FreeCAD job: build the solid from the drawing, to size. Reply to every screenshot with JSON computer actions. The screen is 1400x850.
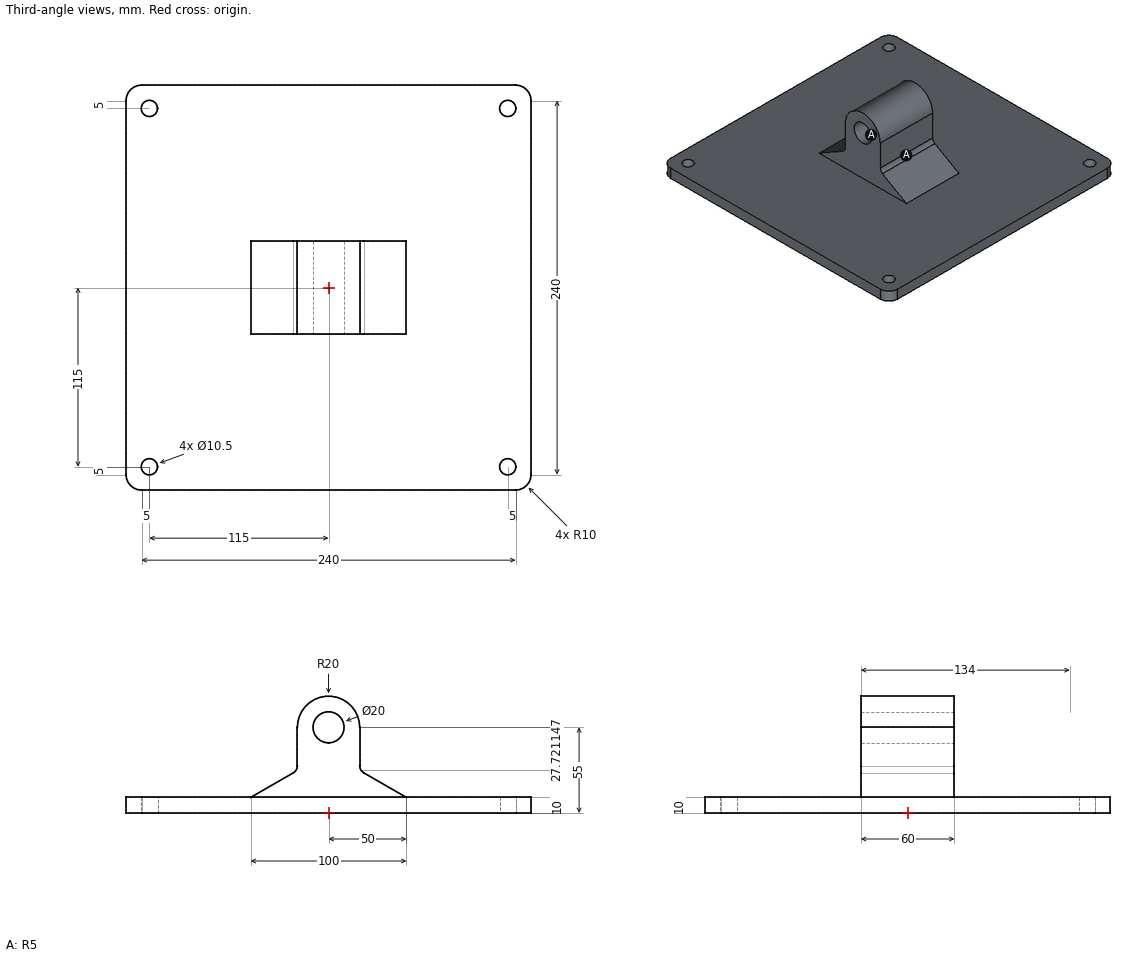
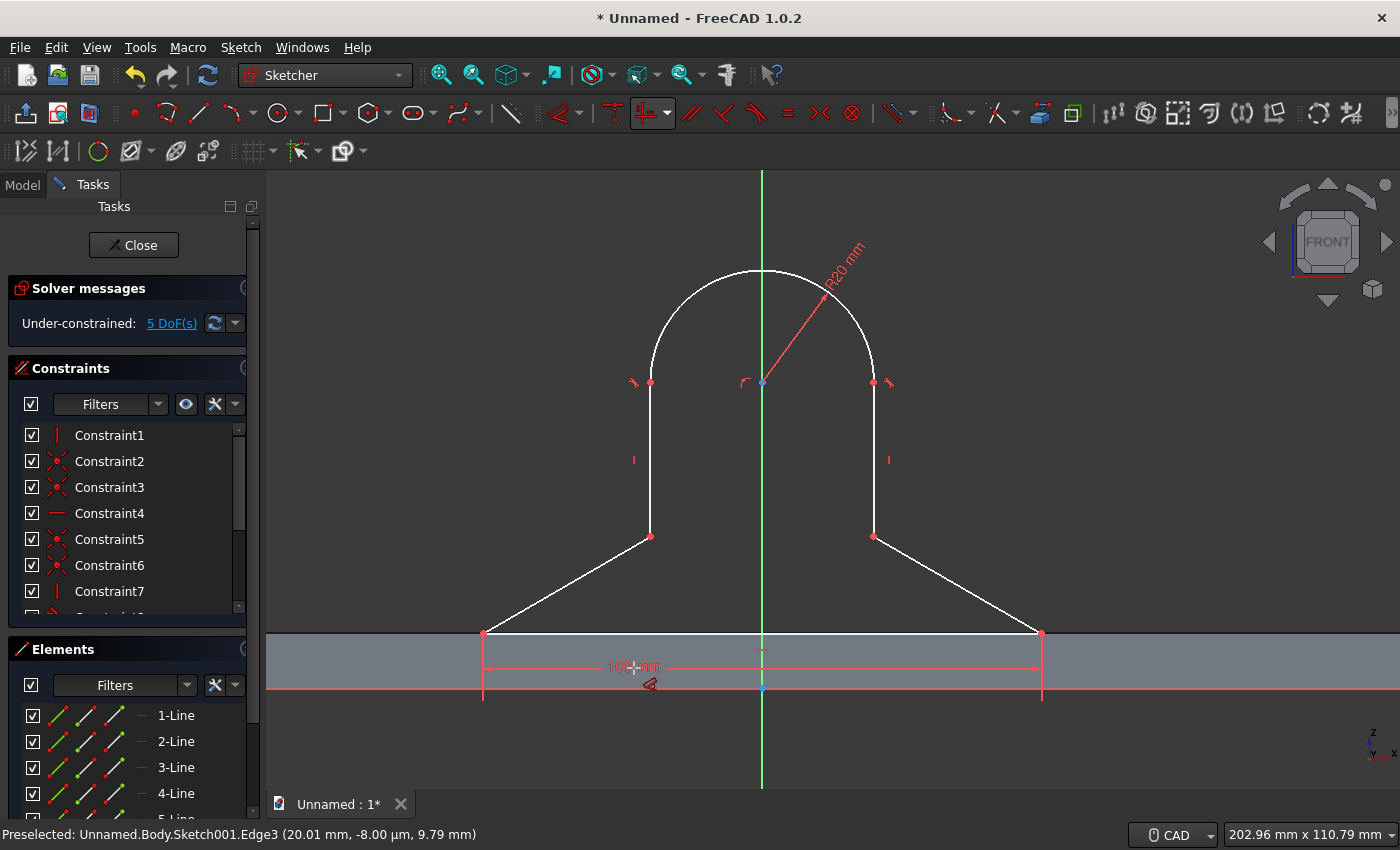
{"action": "left_click", "coordinate": [874, 382]}
{"action": "left_click", "coordinate": [908, 536]}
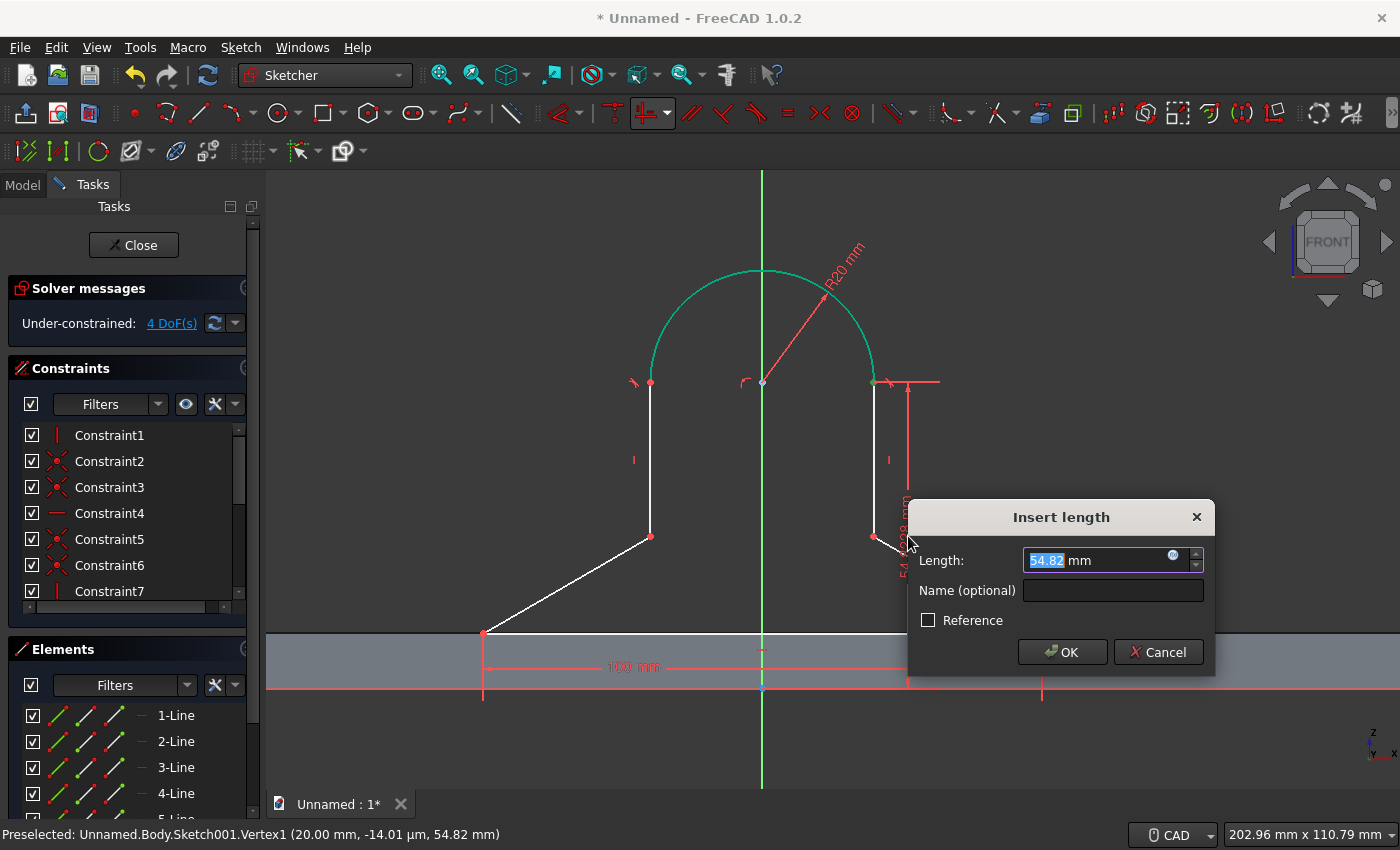
{"action": "type", "text": "55"}
{"action": "key", "text": "Return"}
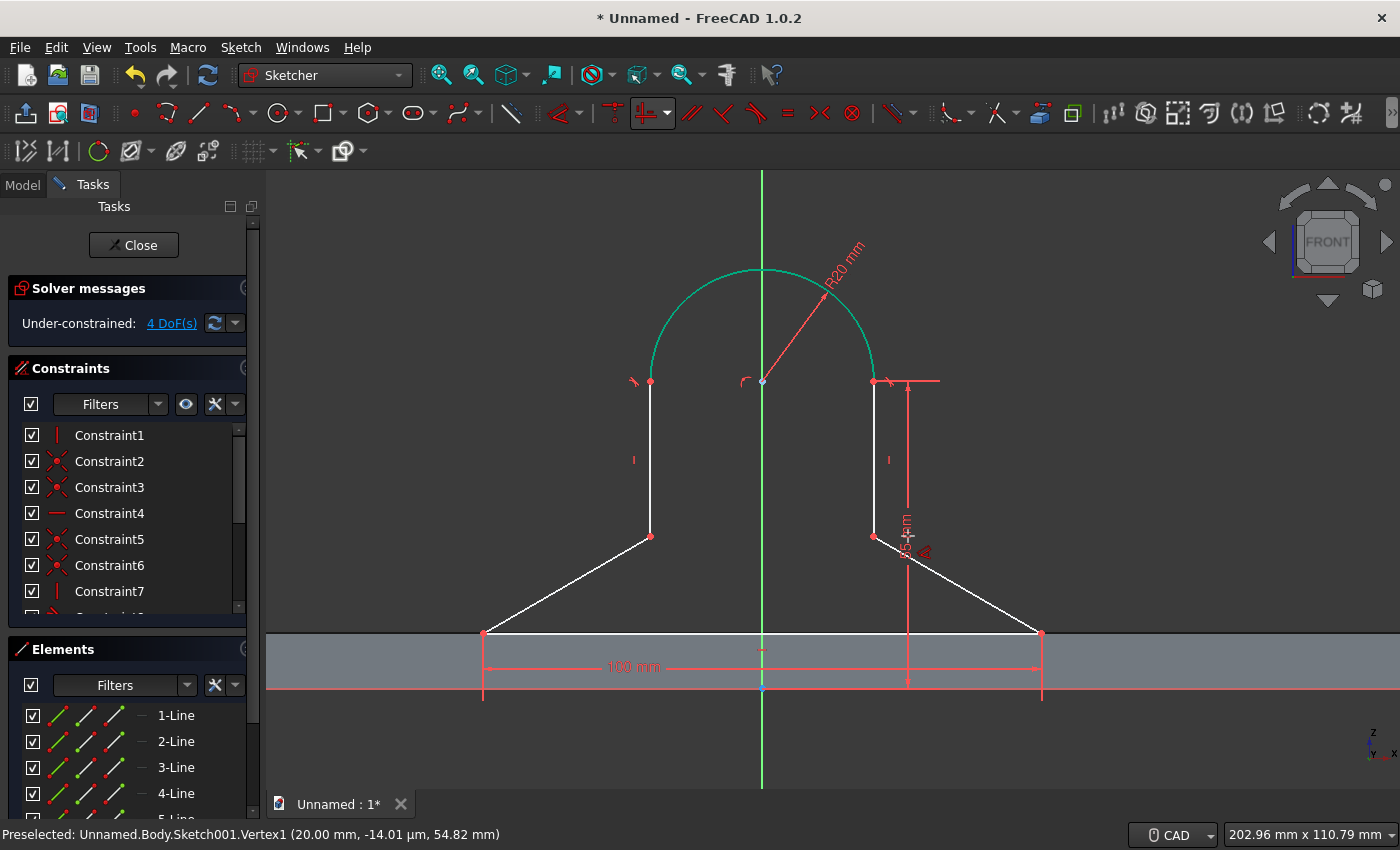
{"action": "left_click", "coordinate": [1042, 634]}
{"action": "left_click", "coordinate": [902, 723]}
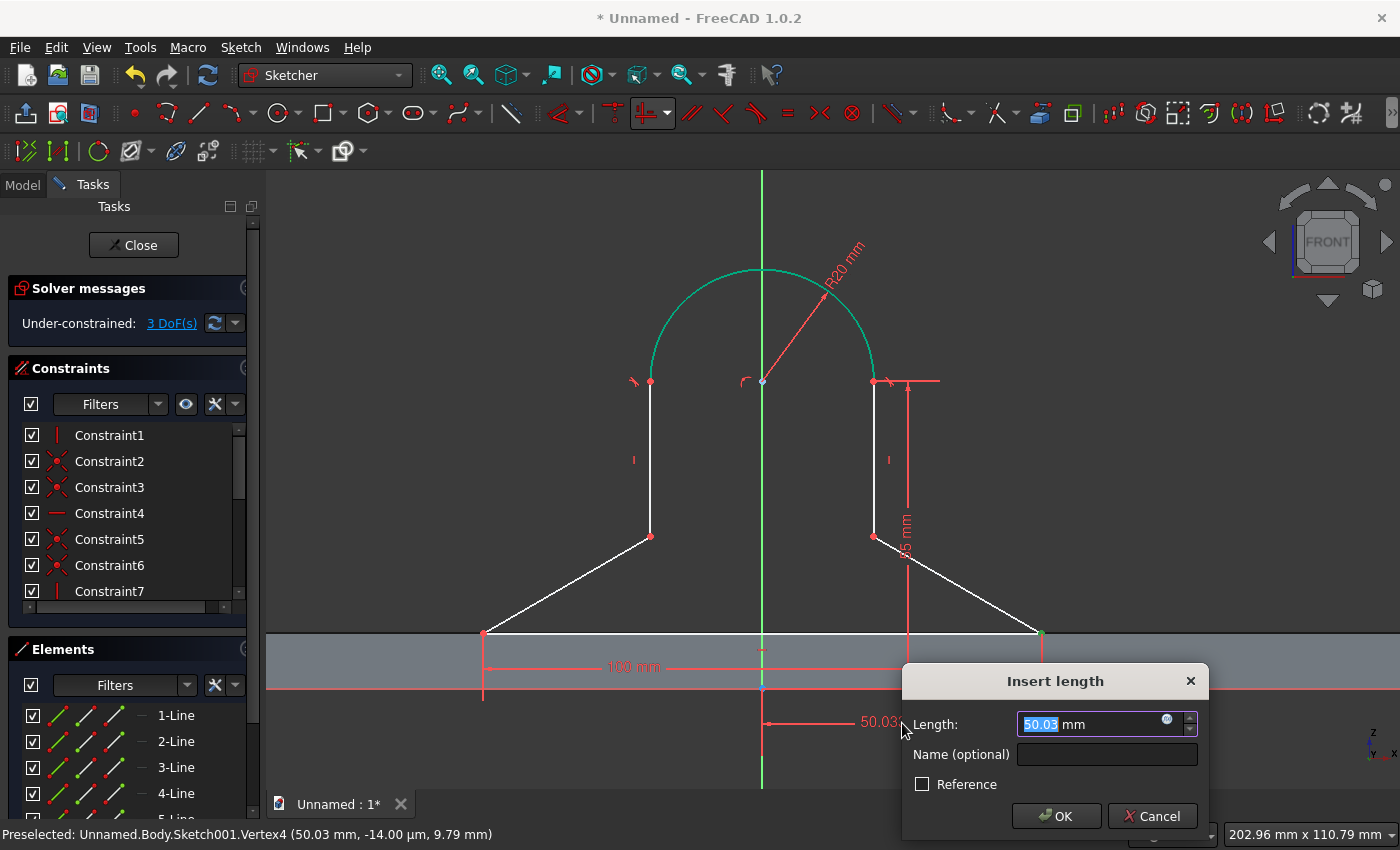
{"action": "type", "text": "50"}
{"action": "key", "text": "Return"}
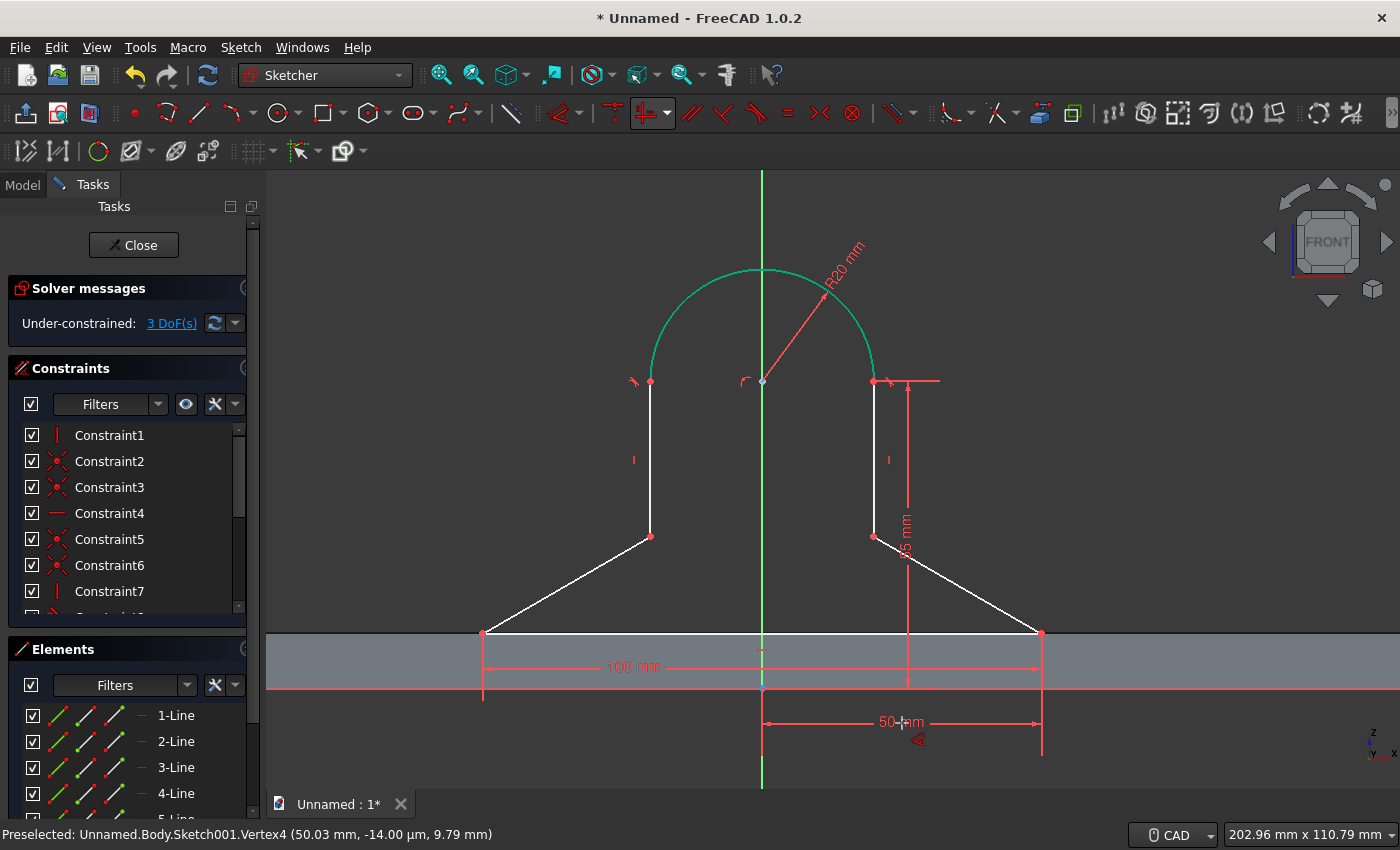
{"action": "left_click", "coordinate": [1042, 634]}
{"action": "left_click", "coordinate": [1076, 661]}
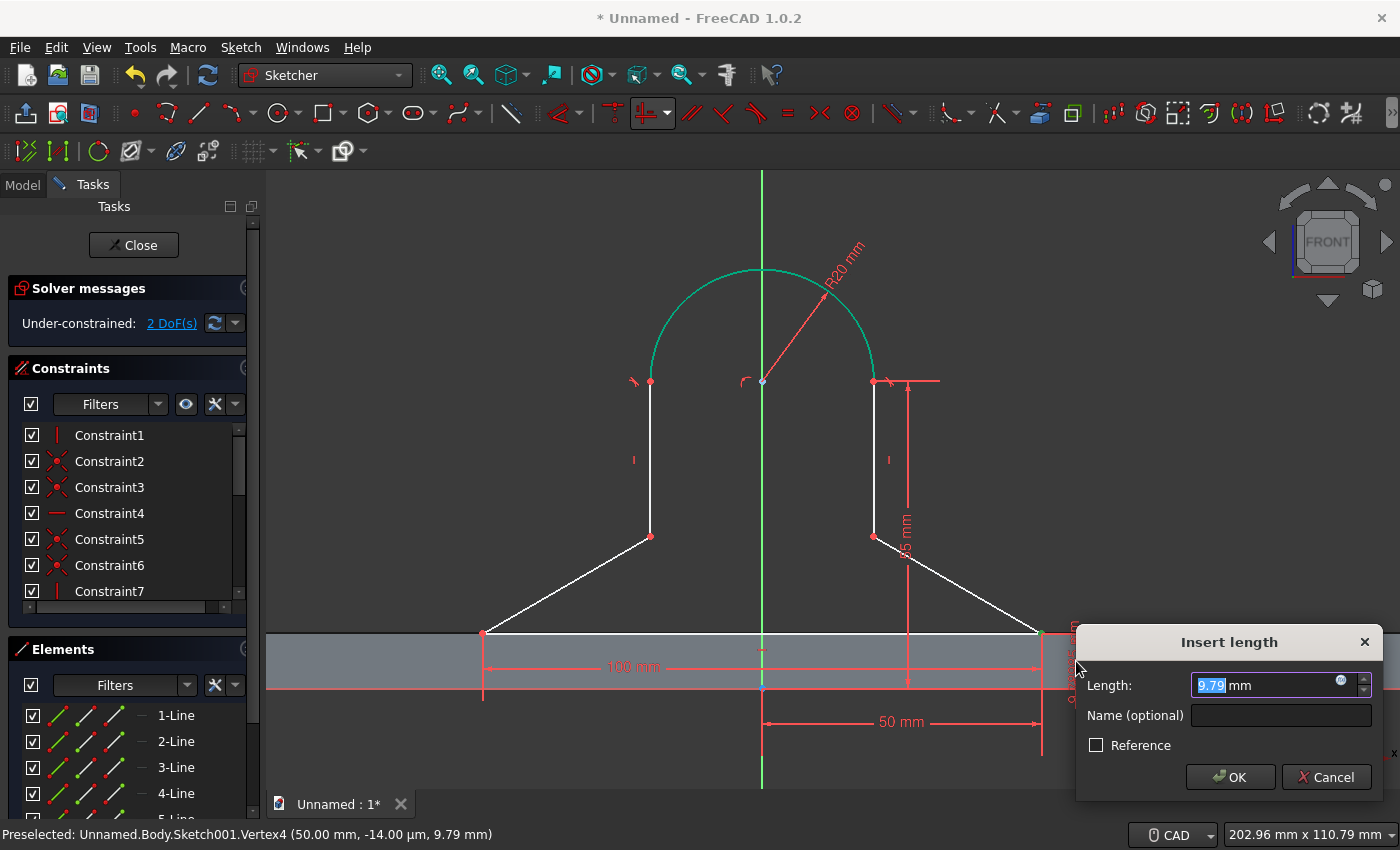
{"action": "type", "text": "10"}
{"action": "key", "text": "Return"}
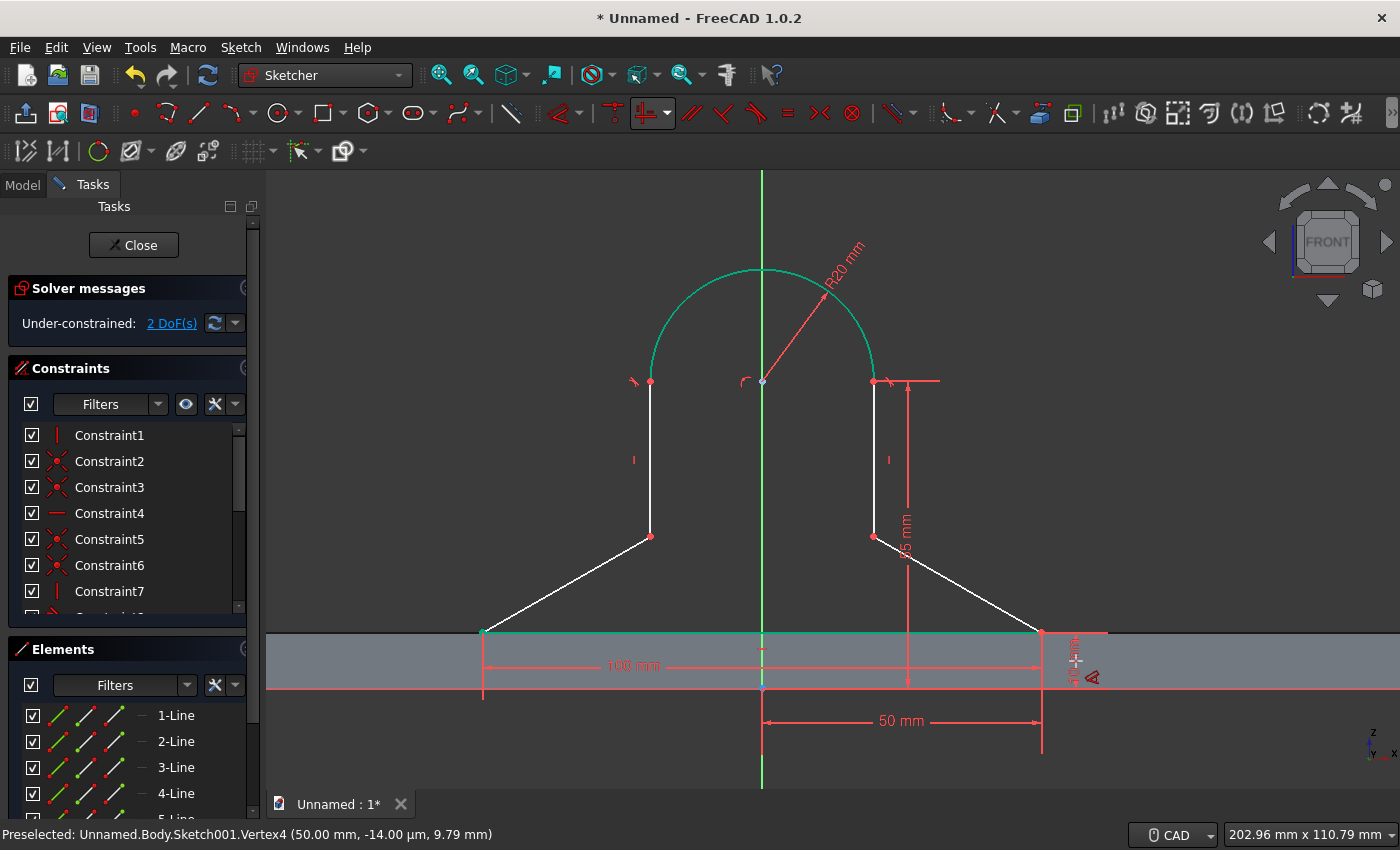
{"action": "left_click", "coordinate": [874, 428]}
{"action": "left_click", "coordinate": [908, 459]}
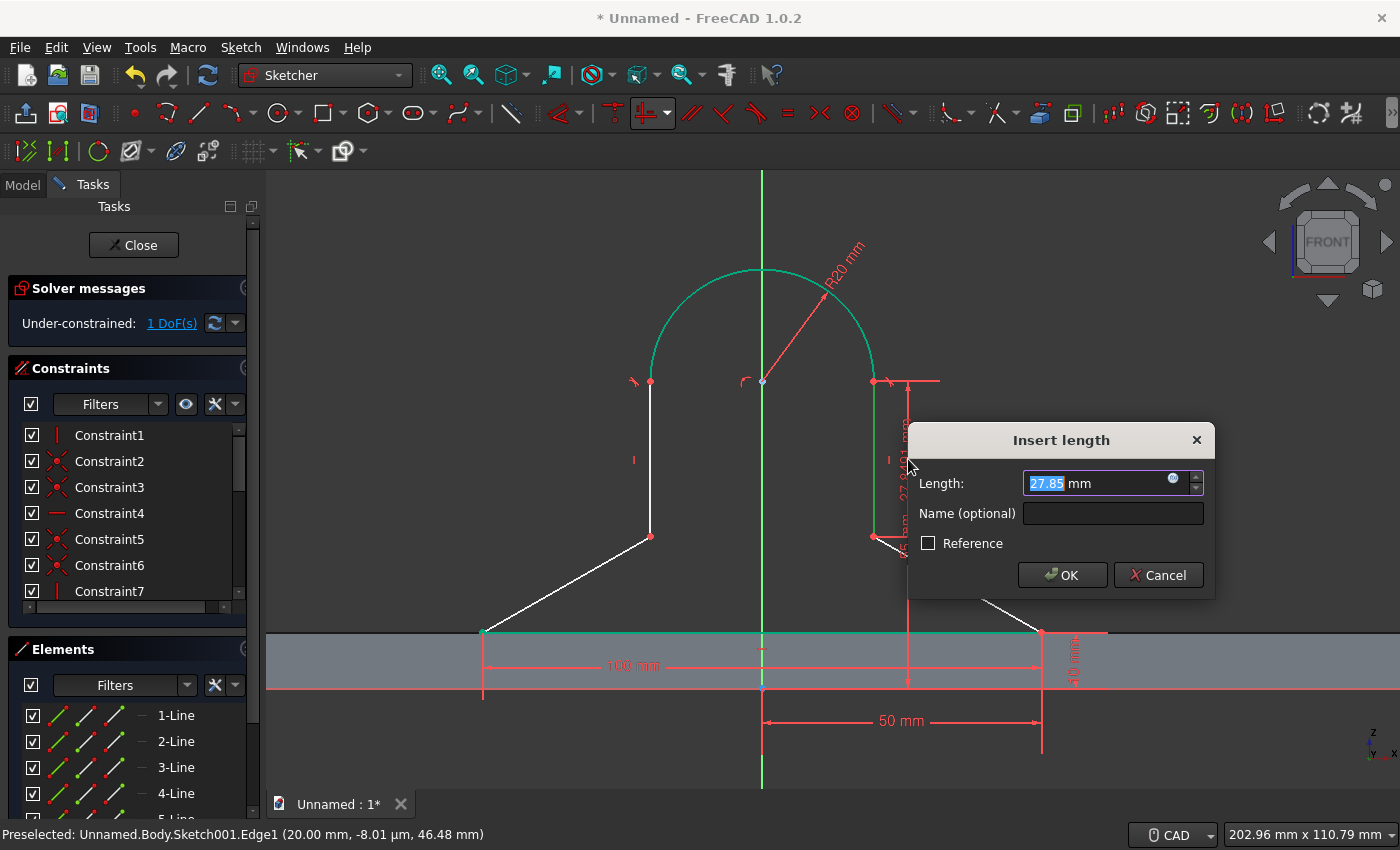
{"action": "type", "text": "27.721147"}
{"action": "key", "text": "Return"}